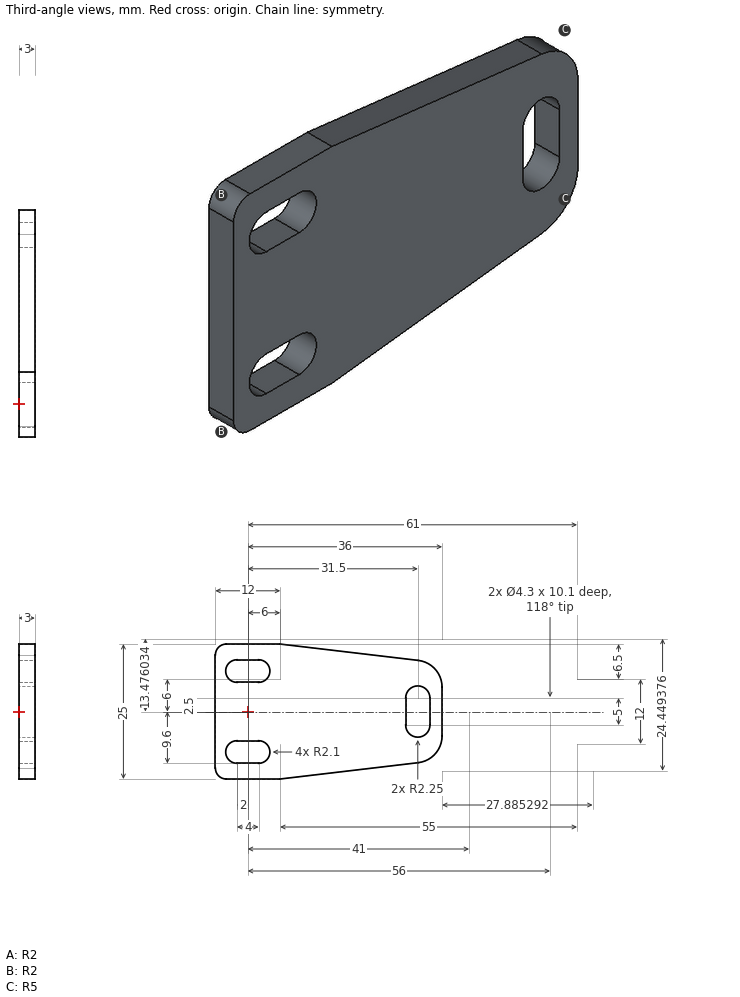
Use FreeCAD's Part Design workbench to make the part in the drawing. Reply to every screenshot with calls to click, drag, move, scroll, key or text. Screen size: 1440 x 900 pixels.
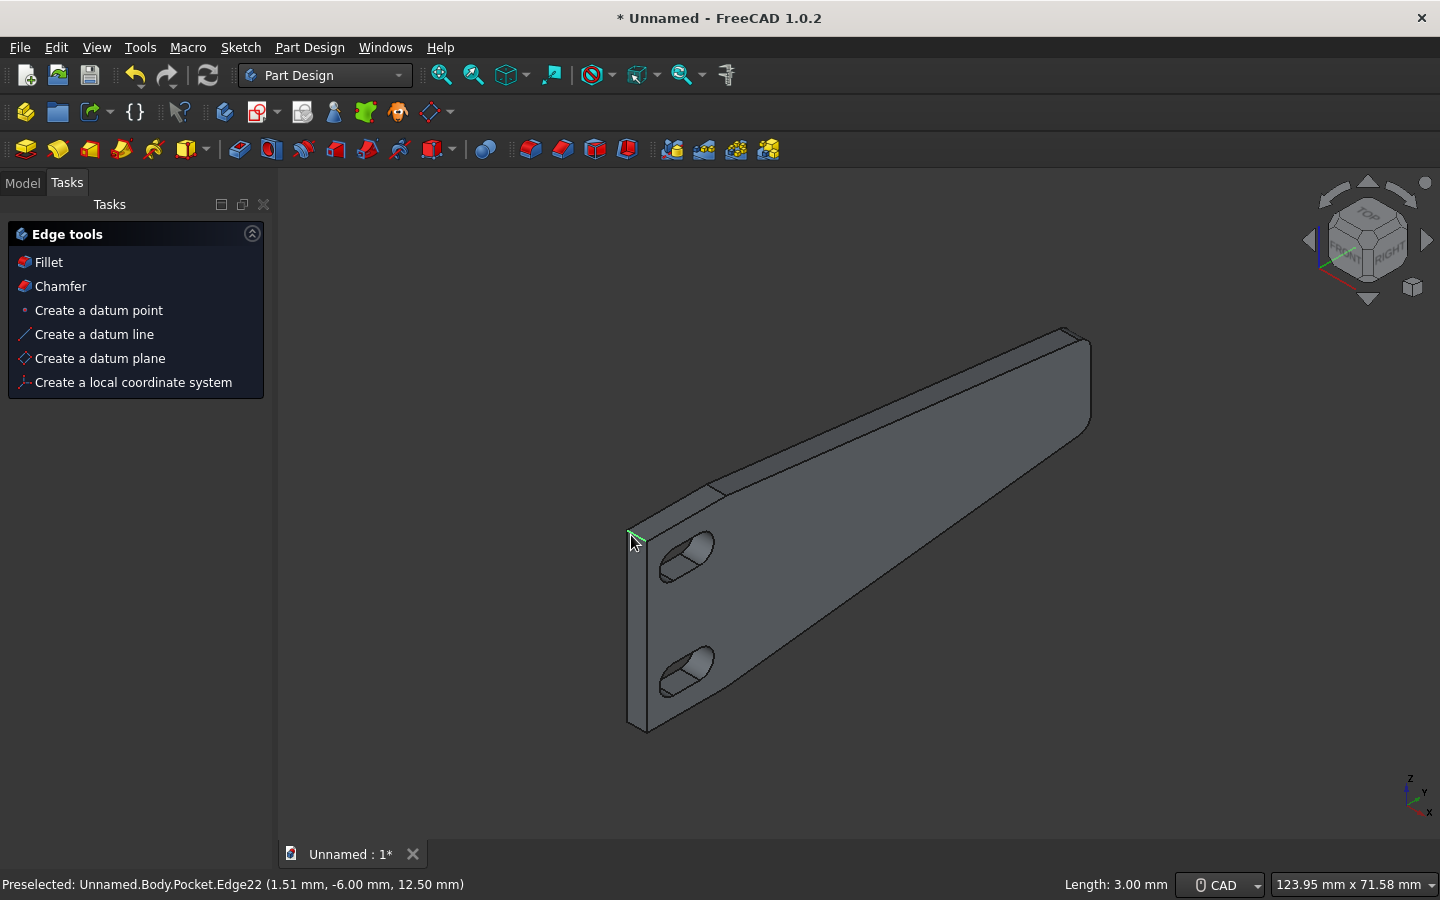
key(2)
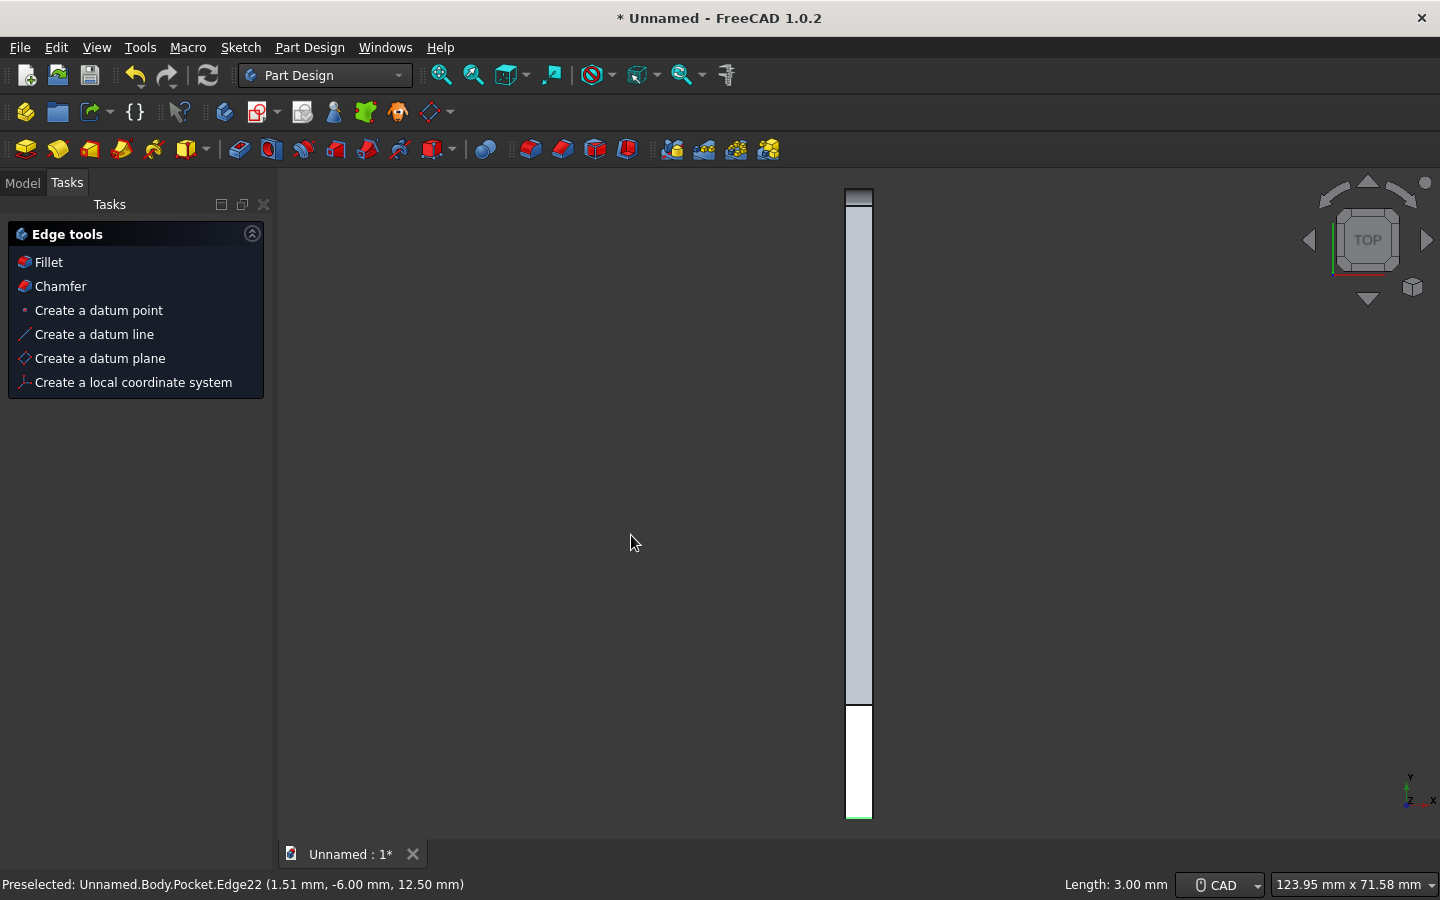
key(1)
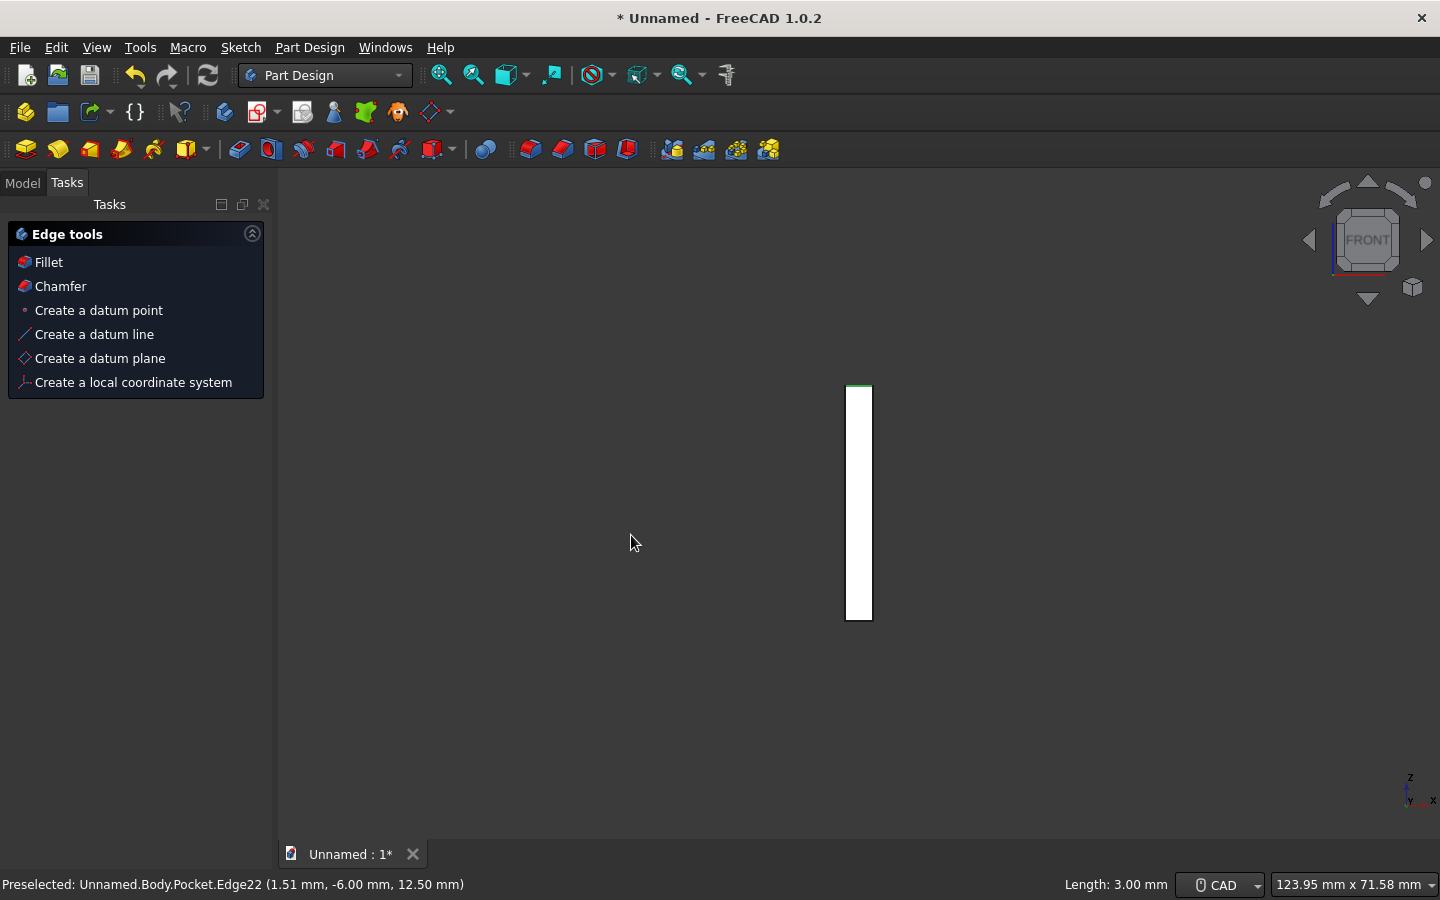
key(v)
key(f)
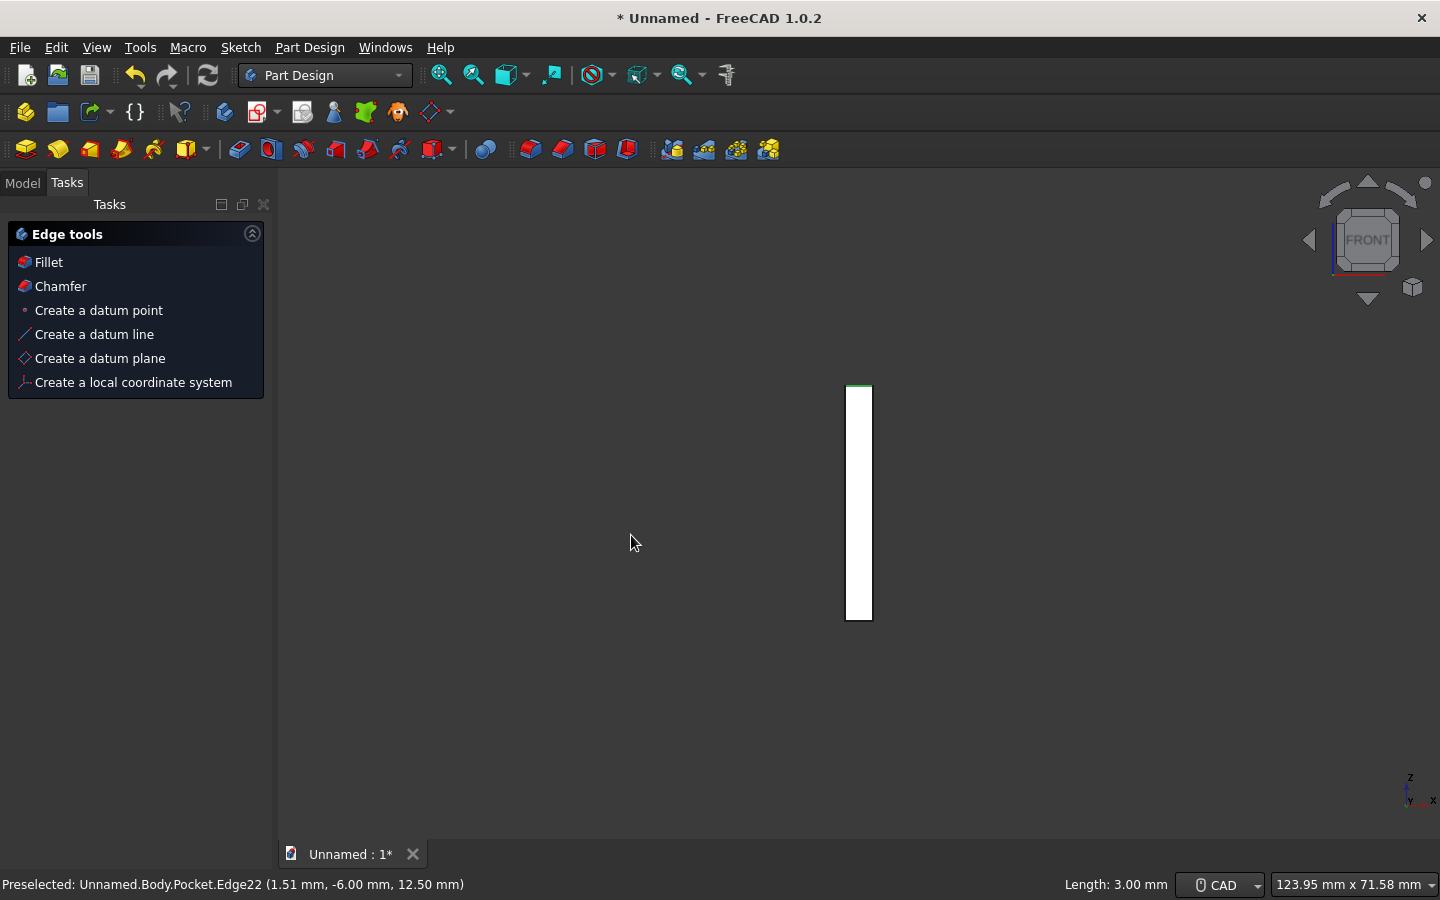
click(859, 620, ctrl)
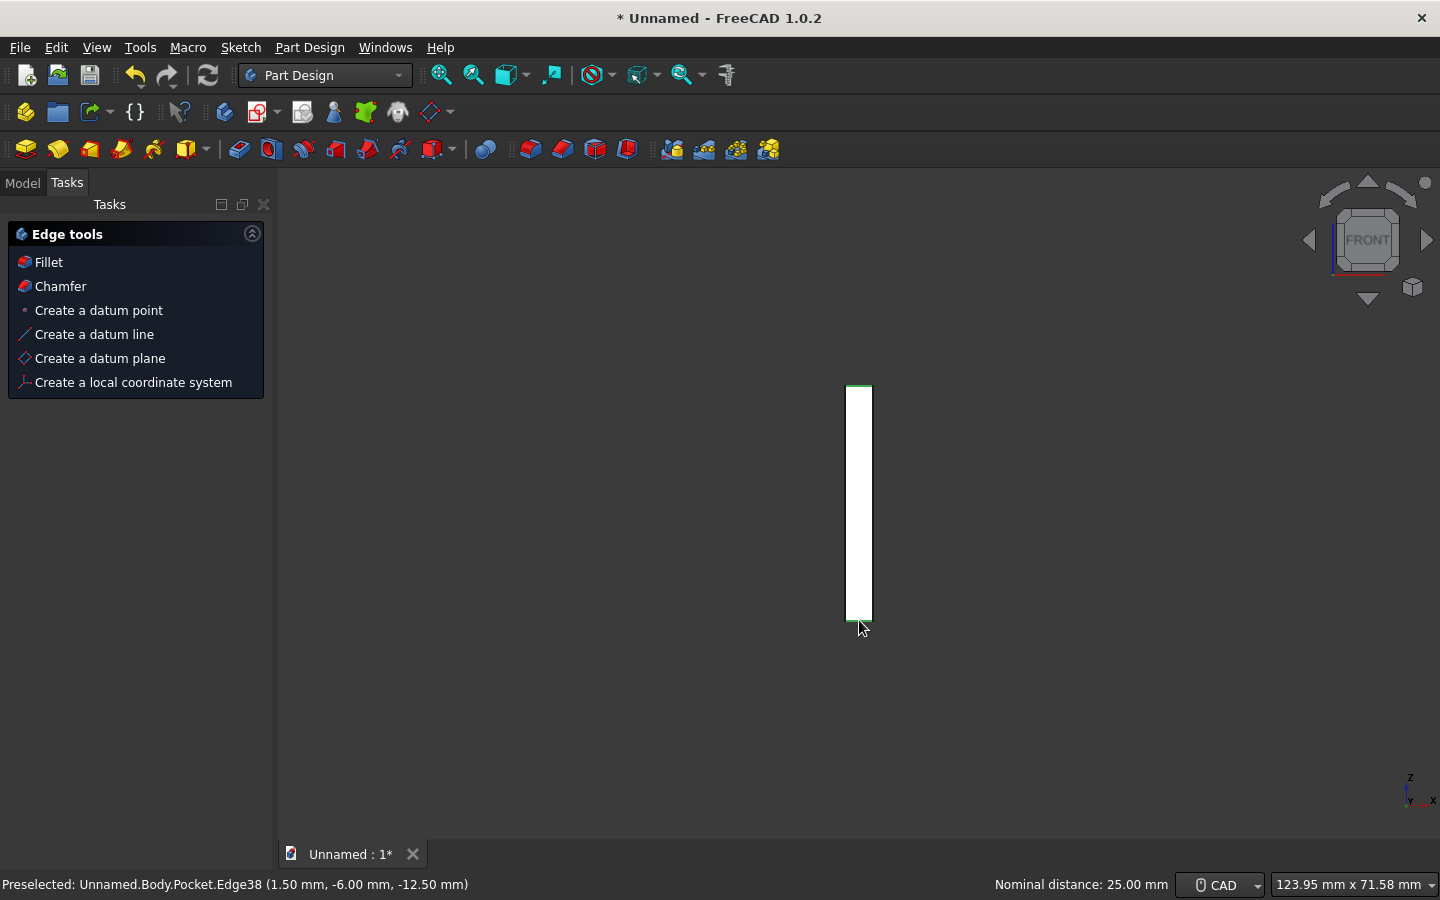
click(532, 150)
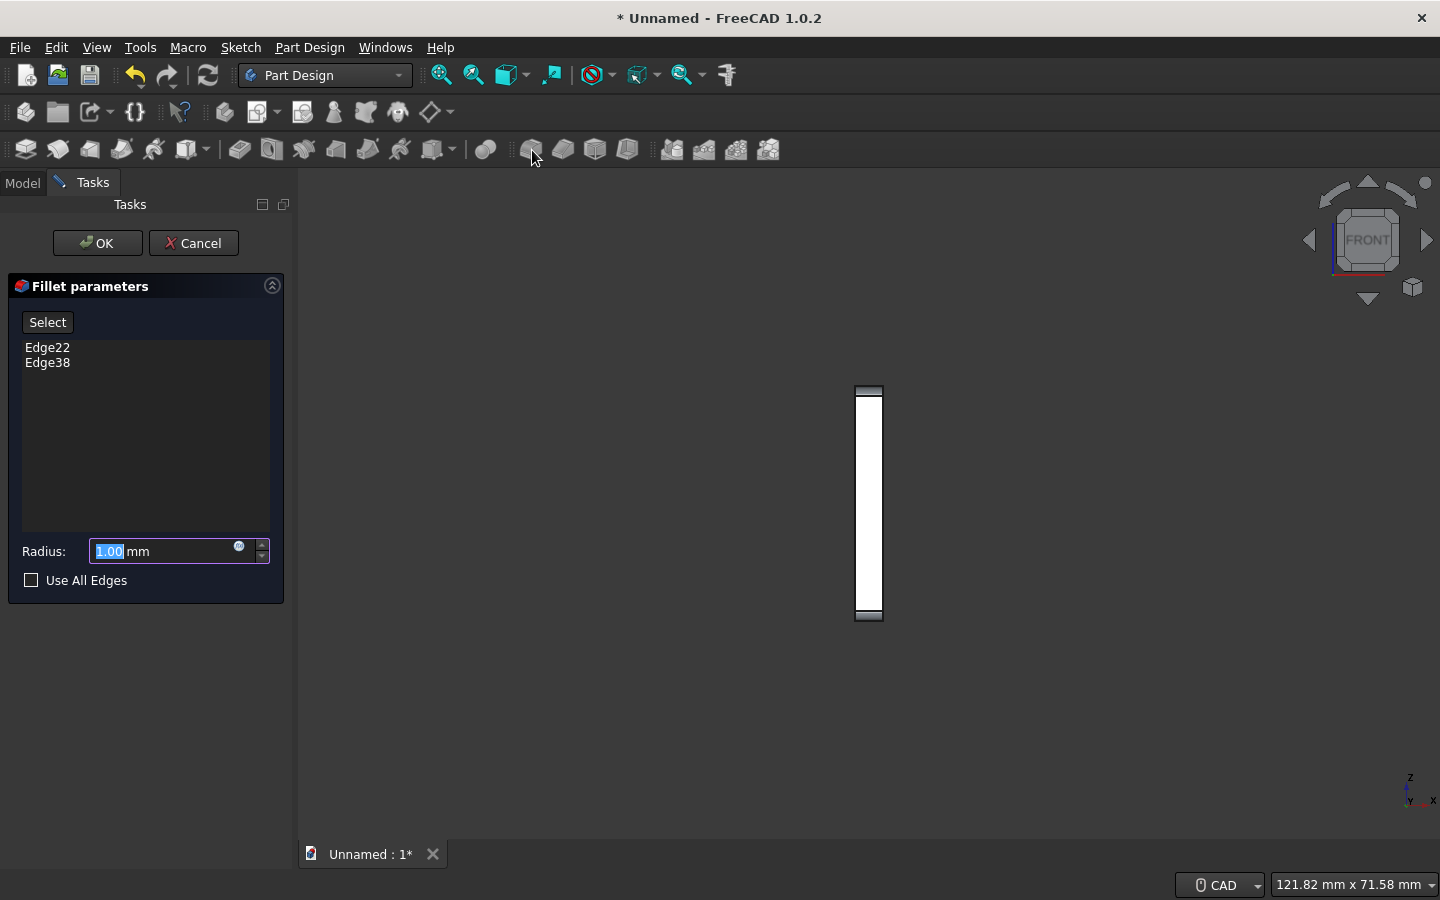
text(2)
key(Tab)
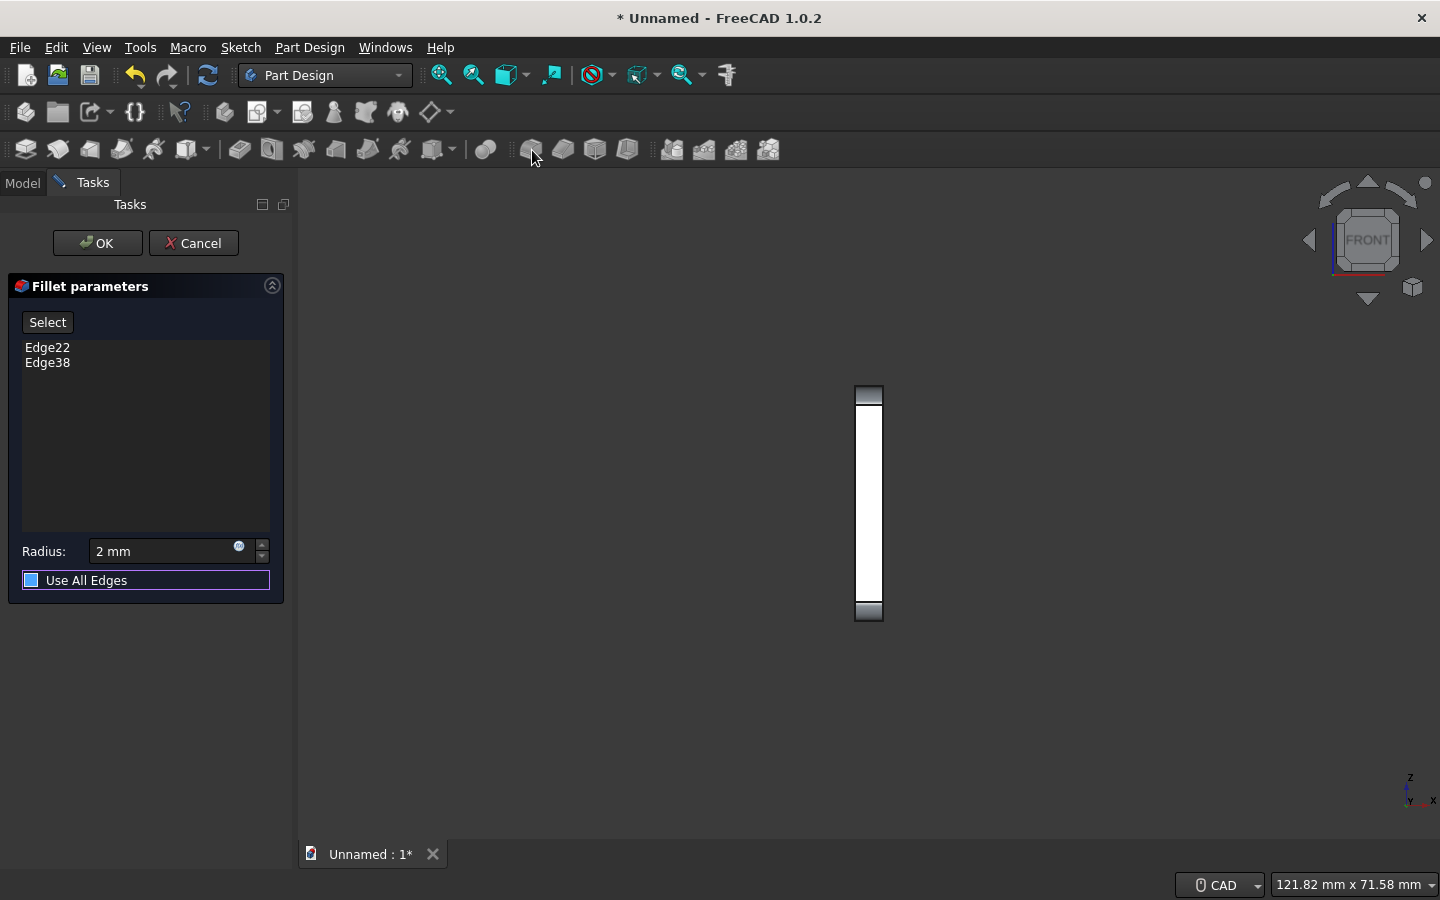
click(98, 243)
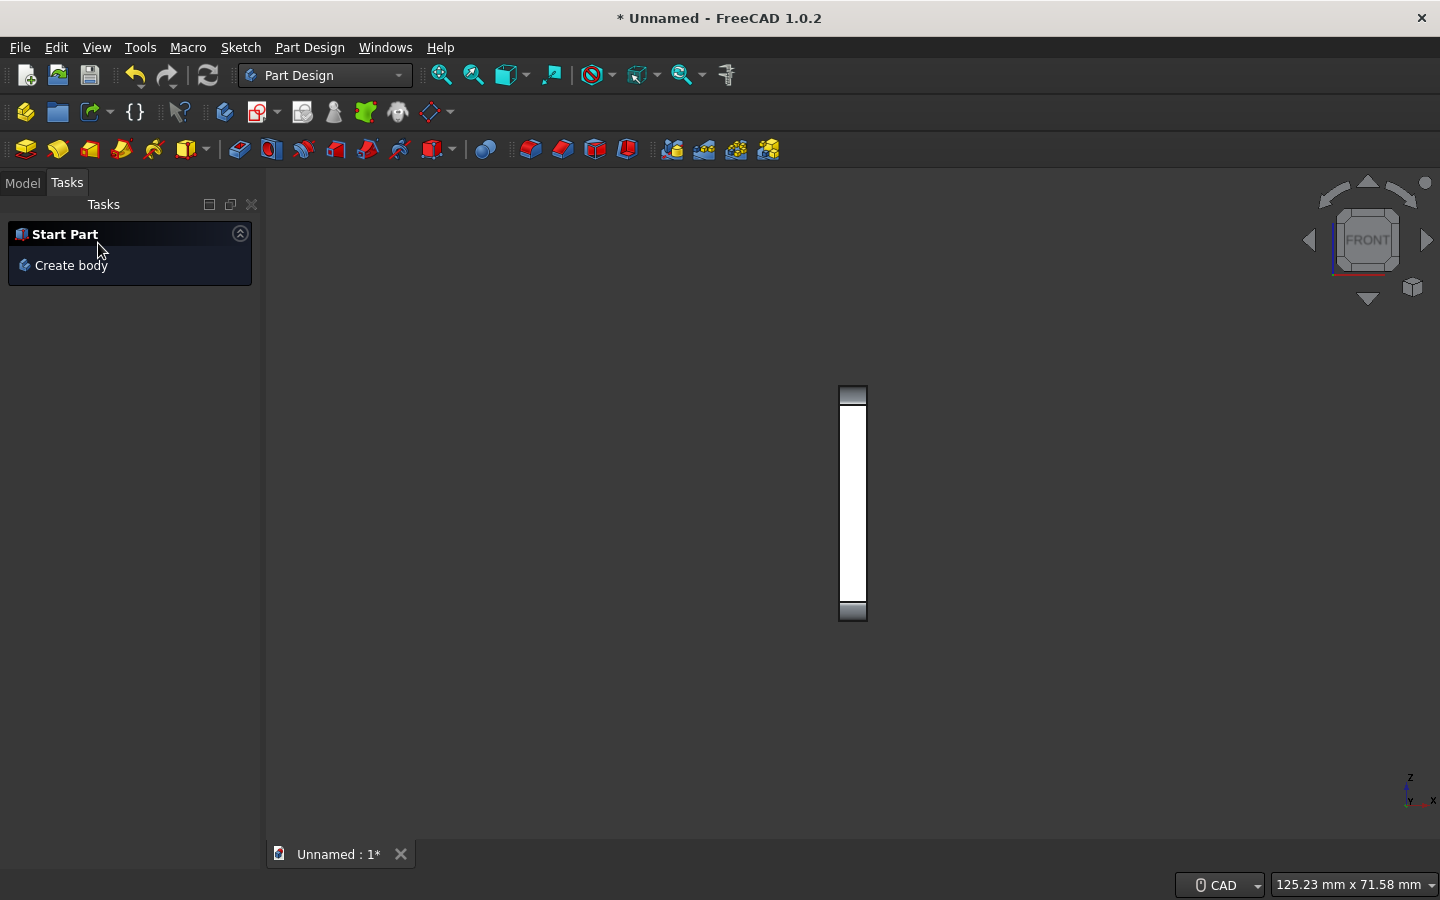
click(442, 76)